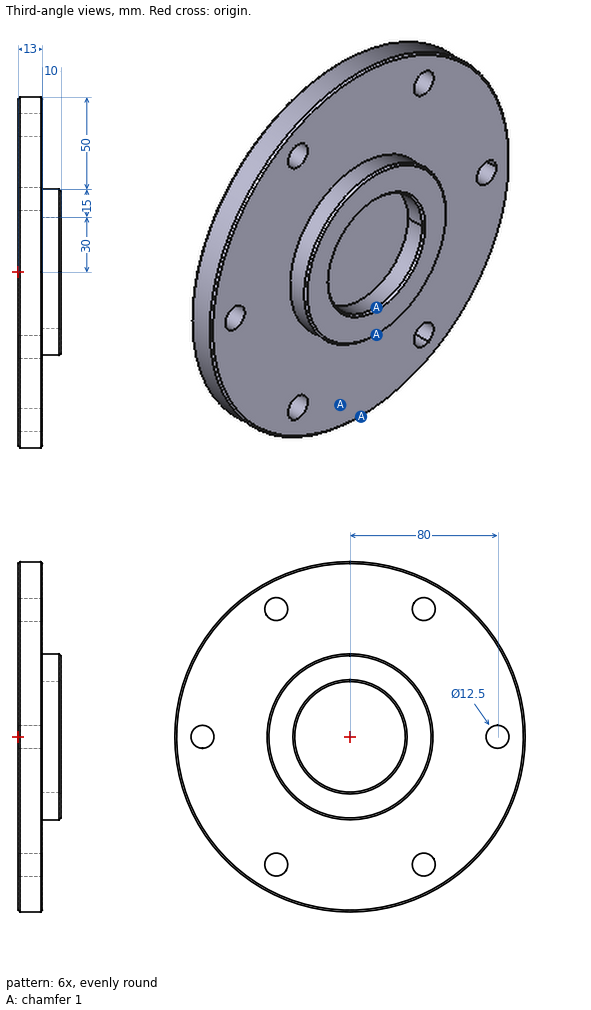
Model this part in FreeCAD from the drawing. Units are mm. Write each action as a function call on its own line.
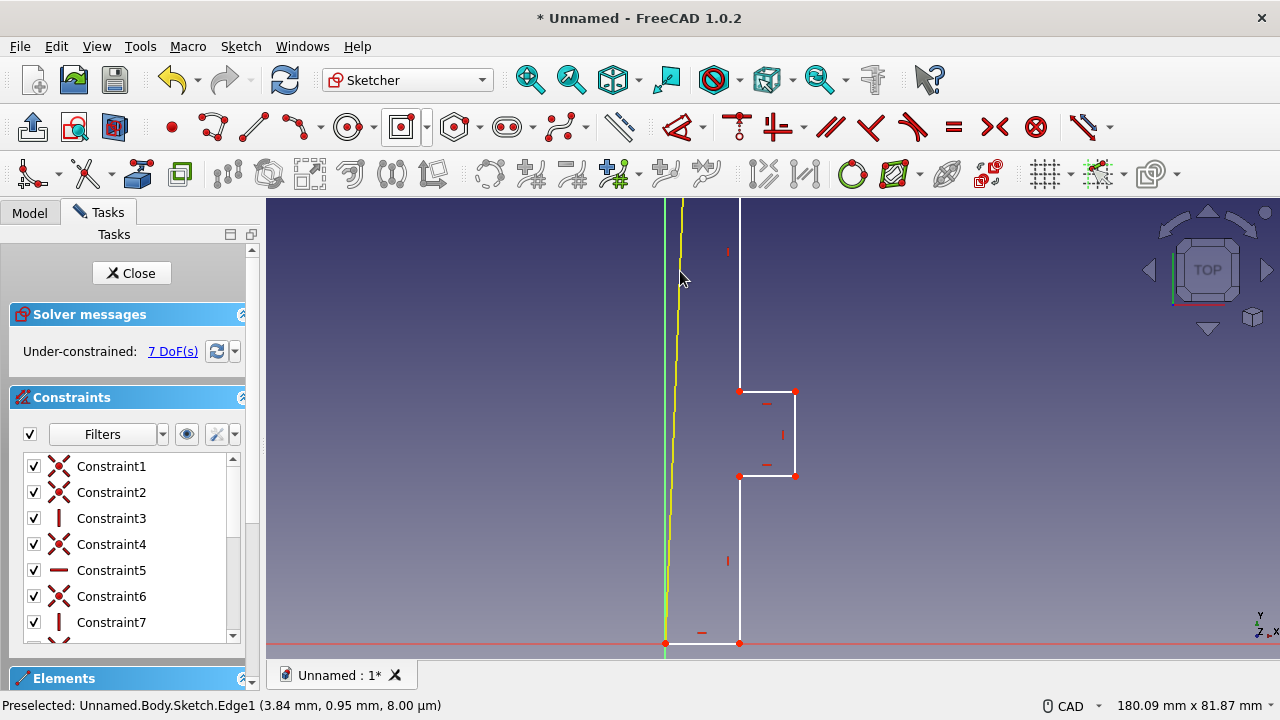
click(680, 271)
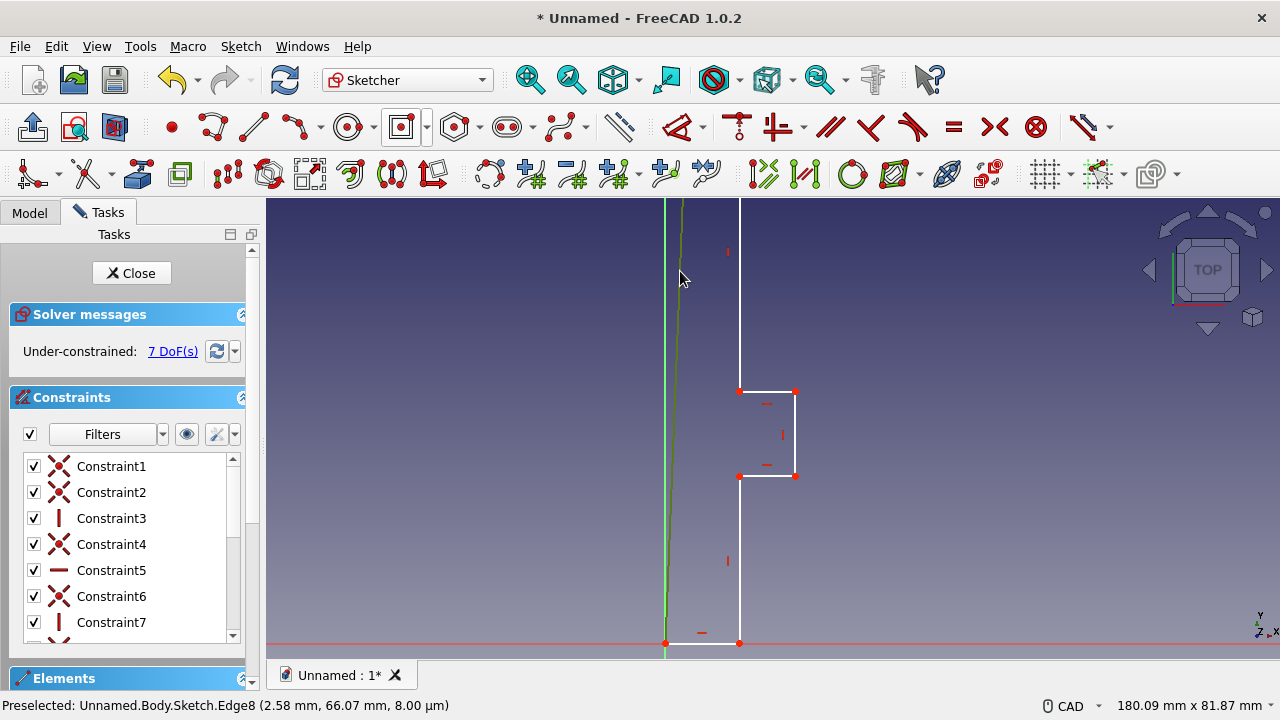
key(v)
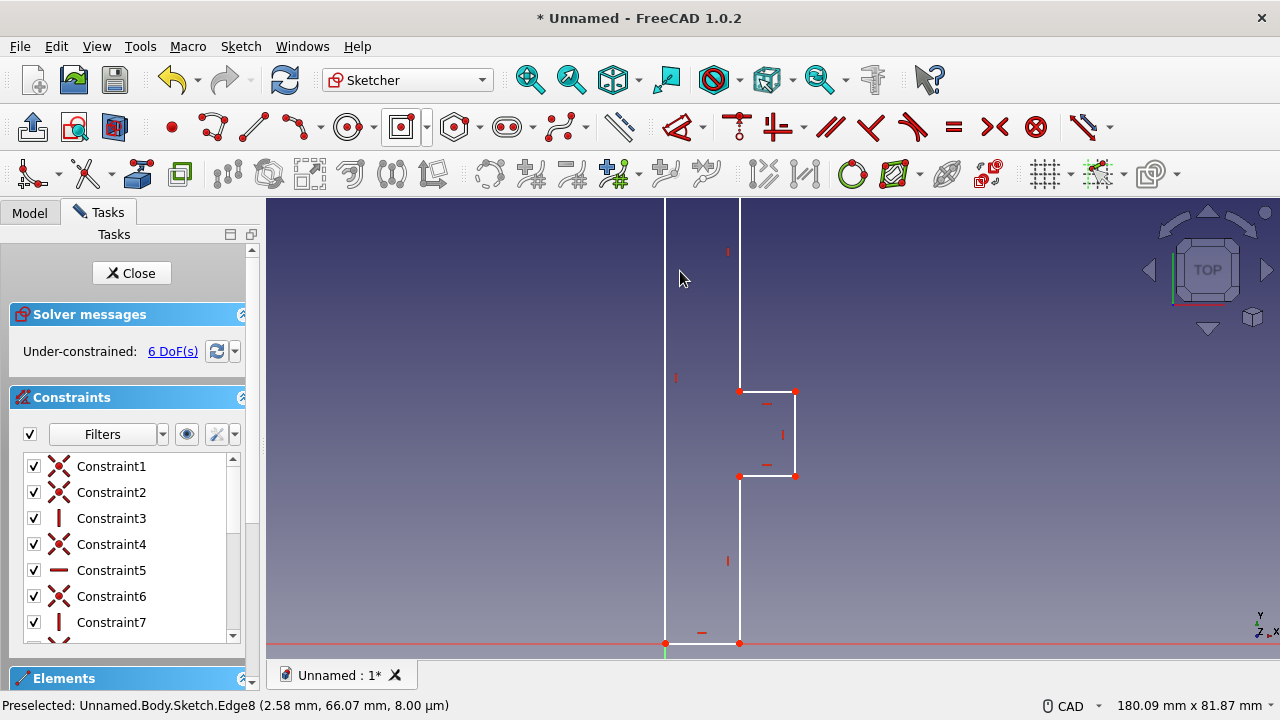
click(676, 128)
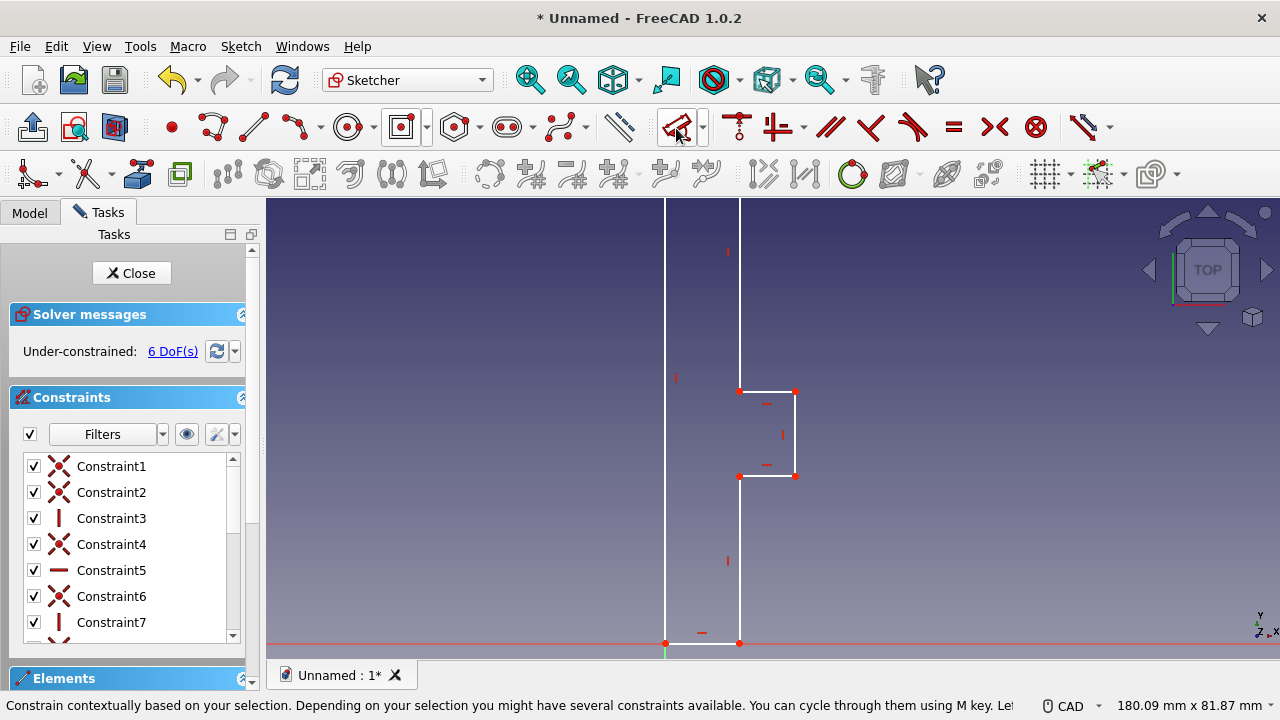
scroll(673, 492, down, 3)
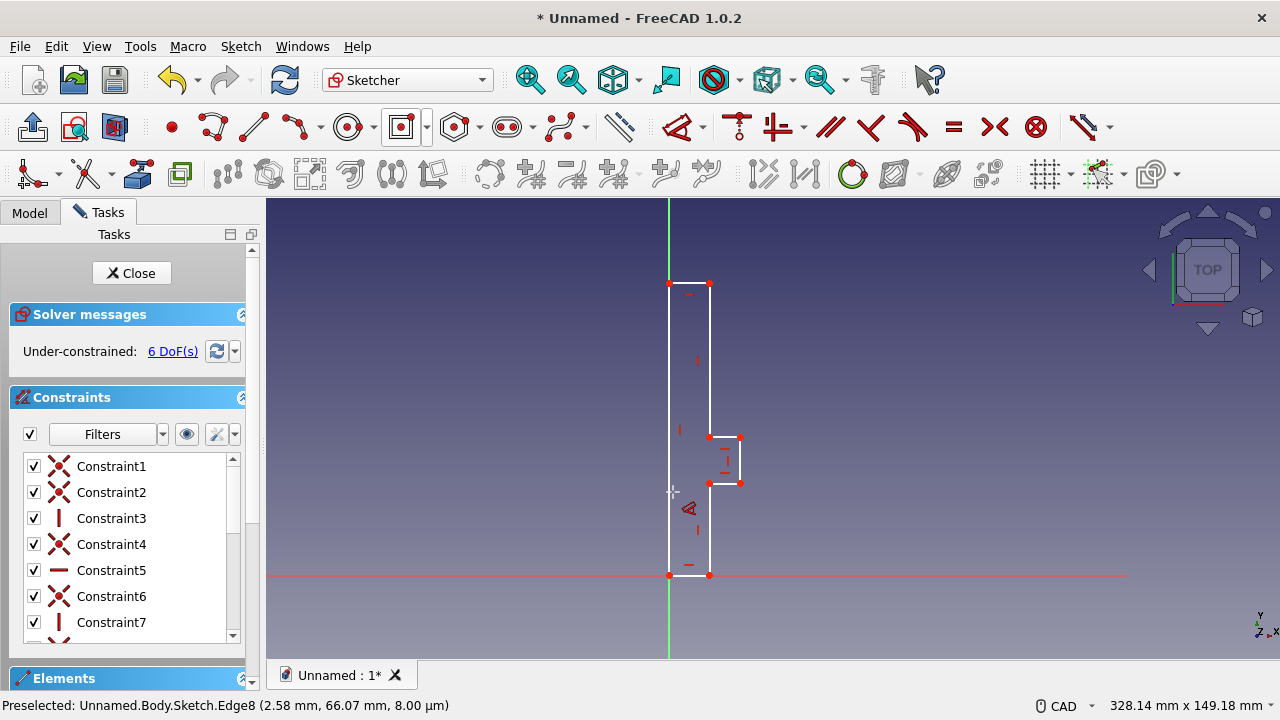
click(681, 576)
click(689, 610)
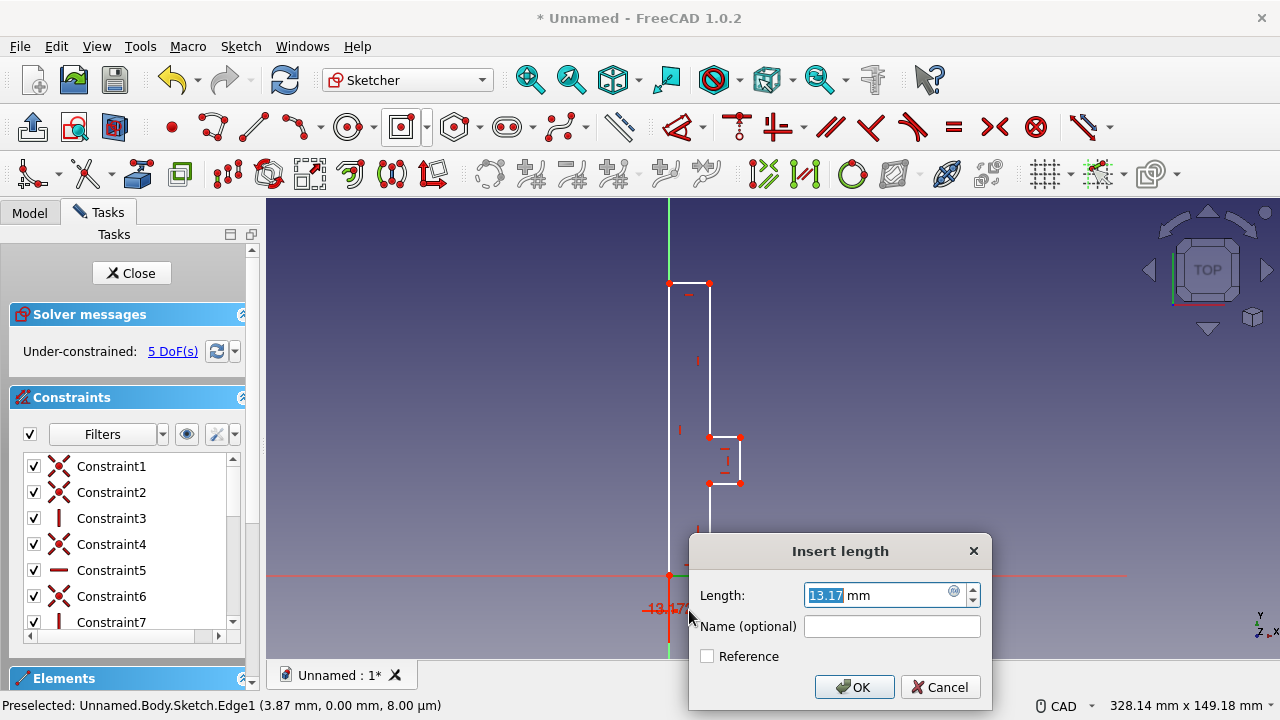
text(13)
key(Return)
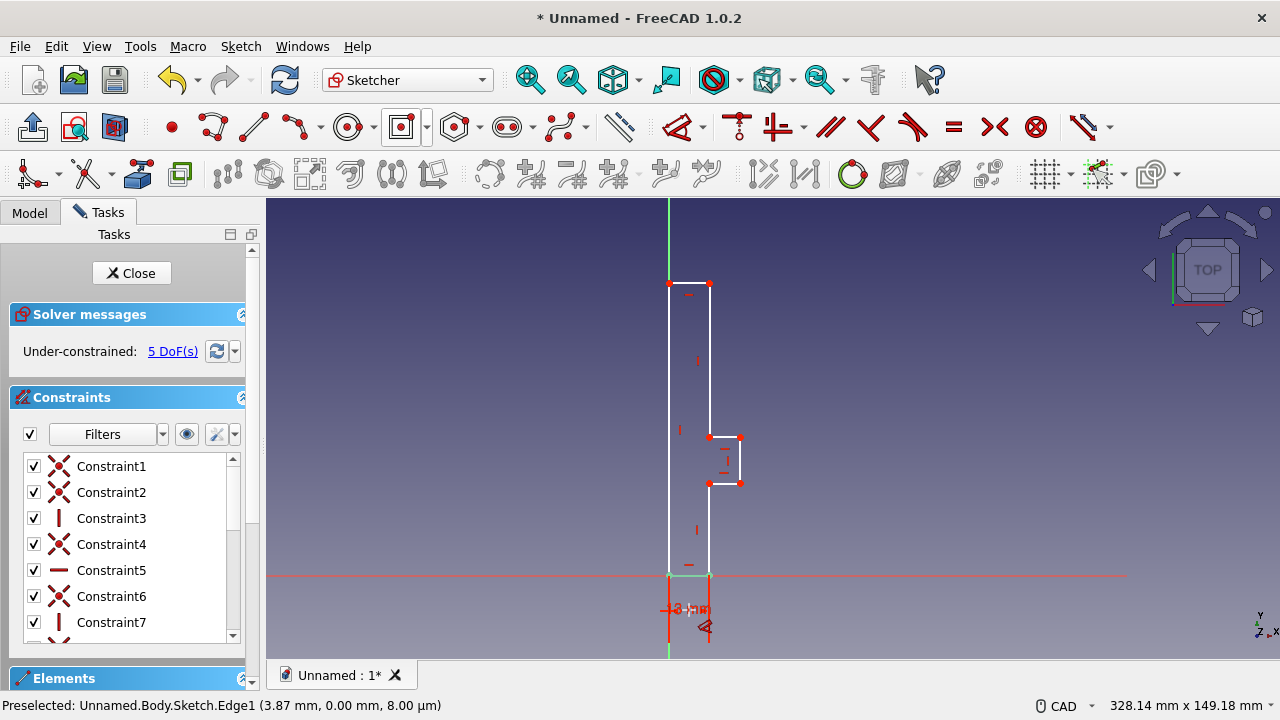
click(709, 548)
click(743, 530)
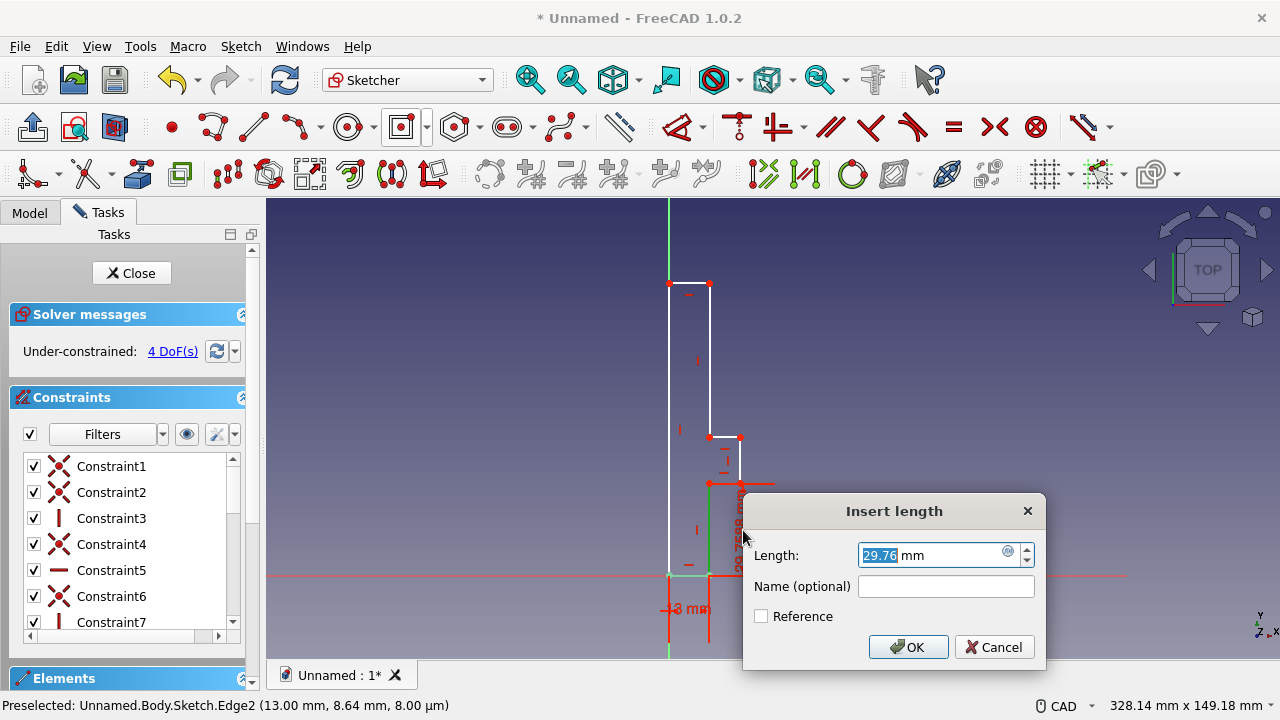
text(30)
key(Return)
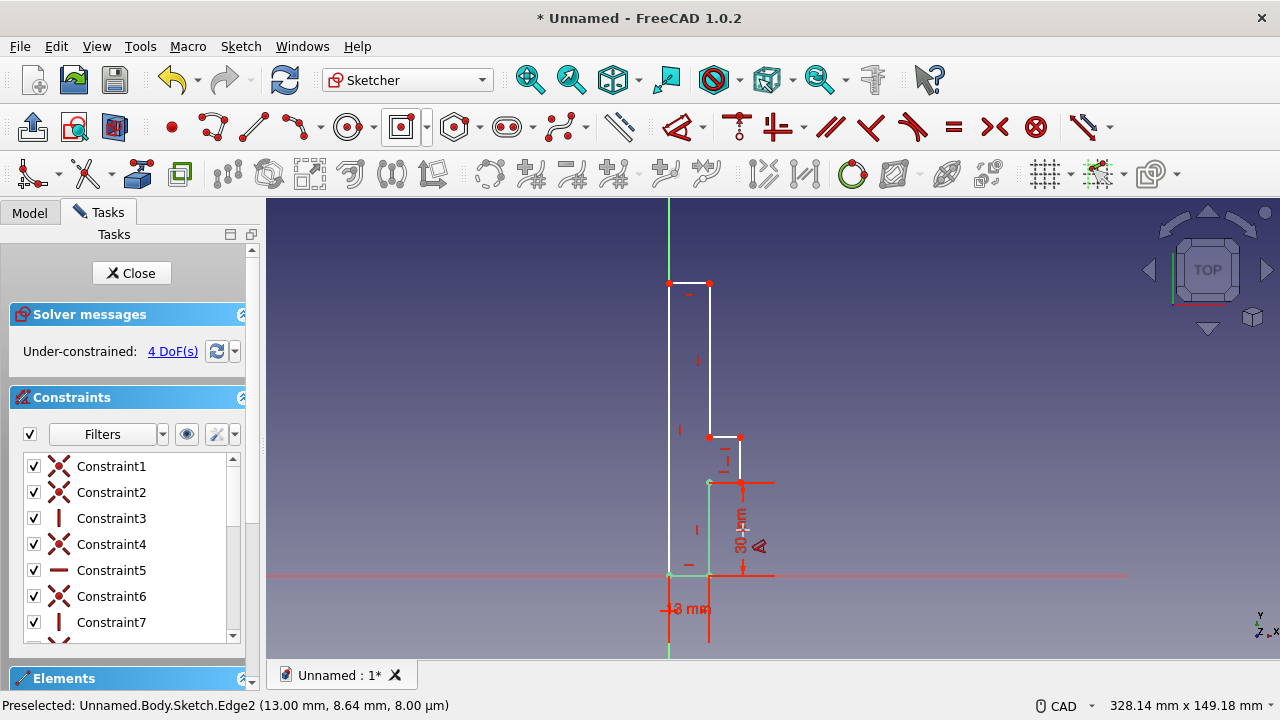
scroll(719, 483, up, 2)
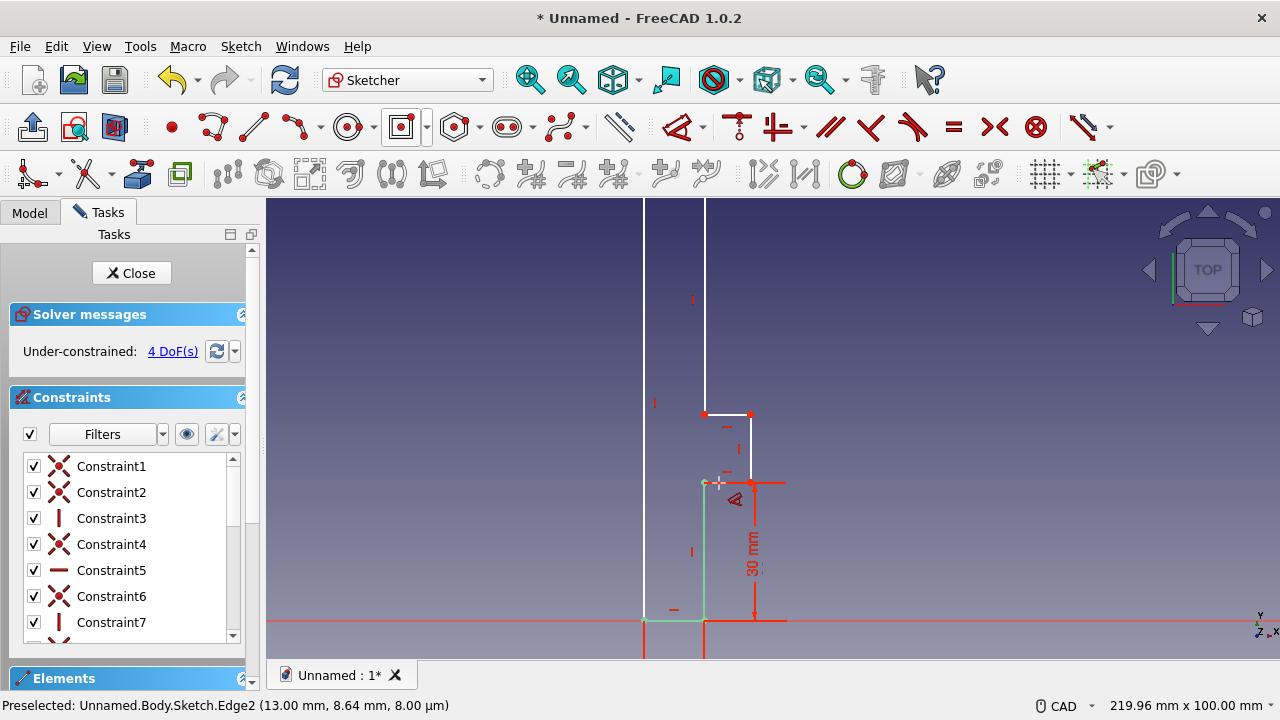
click(718, 483)
click(727, 517)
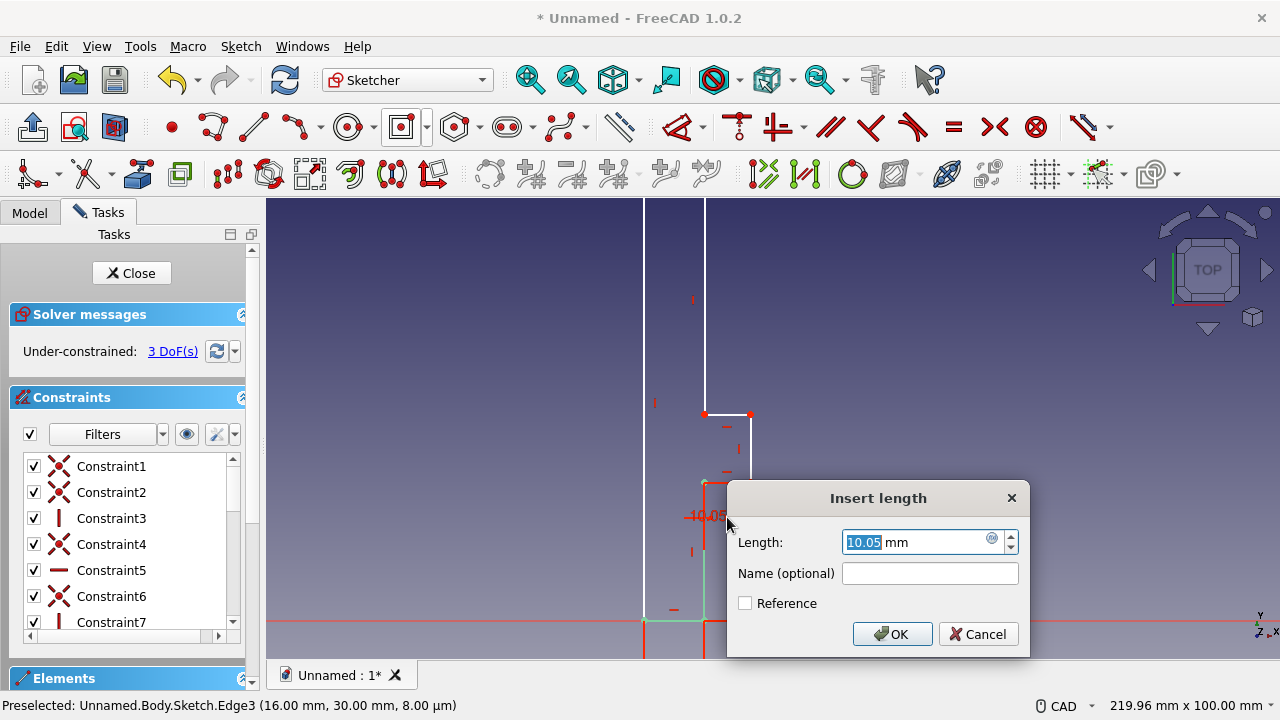
text(10)
key(Return)